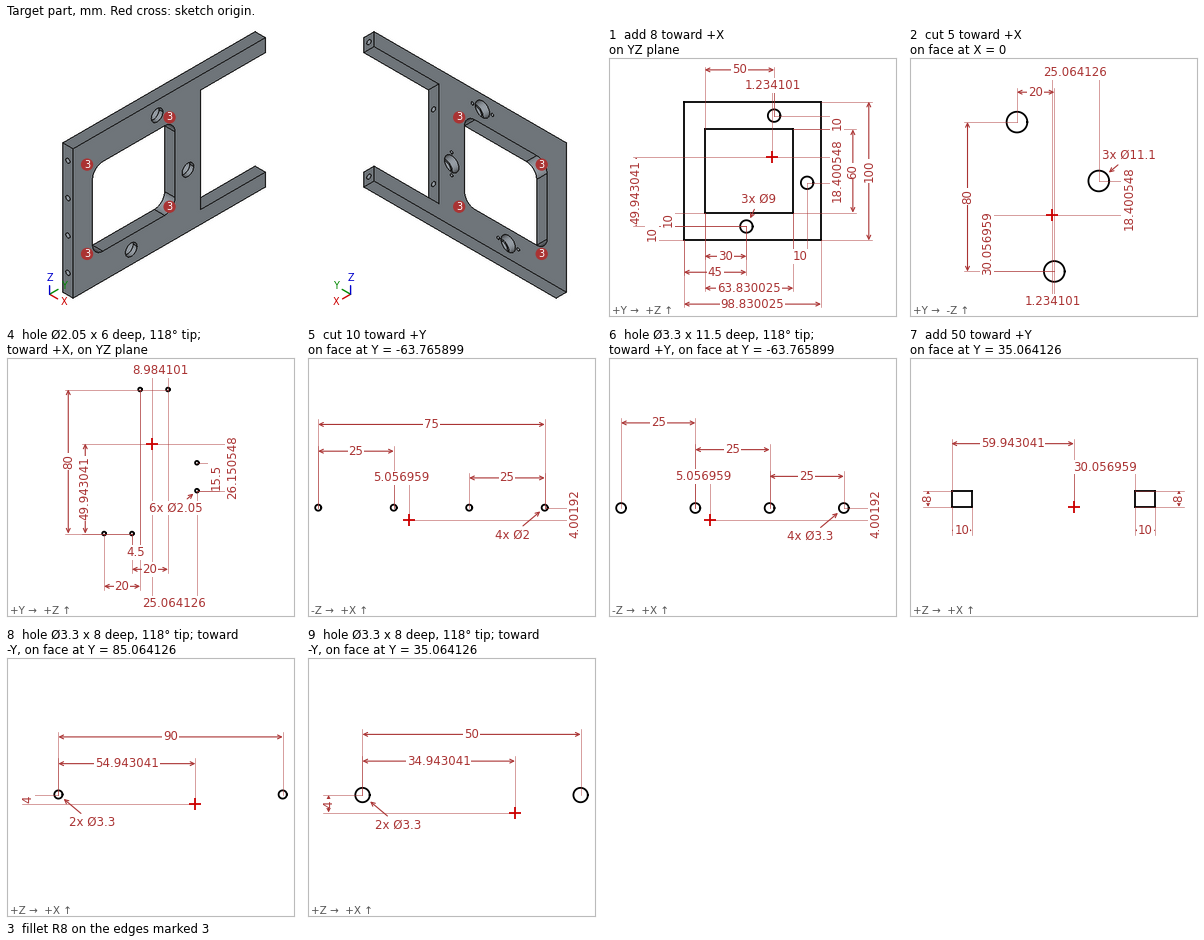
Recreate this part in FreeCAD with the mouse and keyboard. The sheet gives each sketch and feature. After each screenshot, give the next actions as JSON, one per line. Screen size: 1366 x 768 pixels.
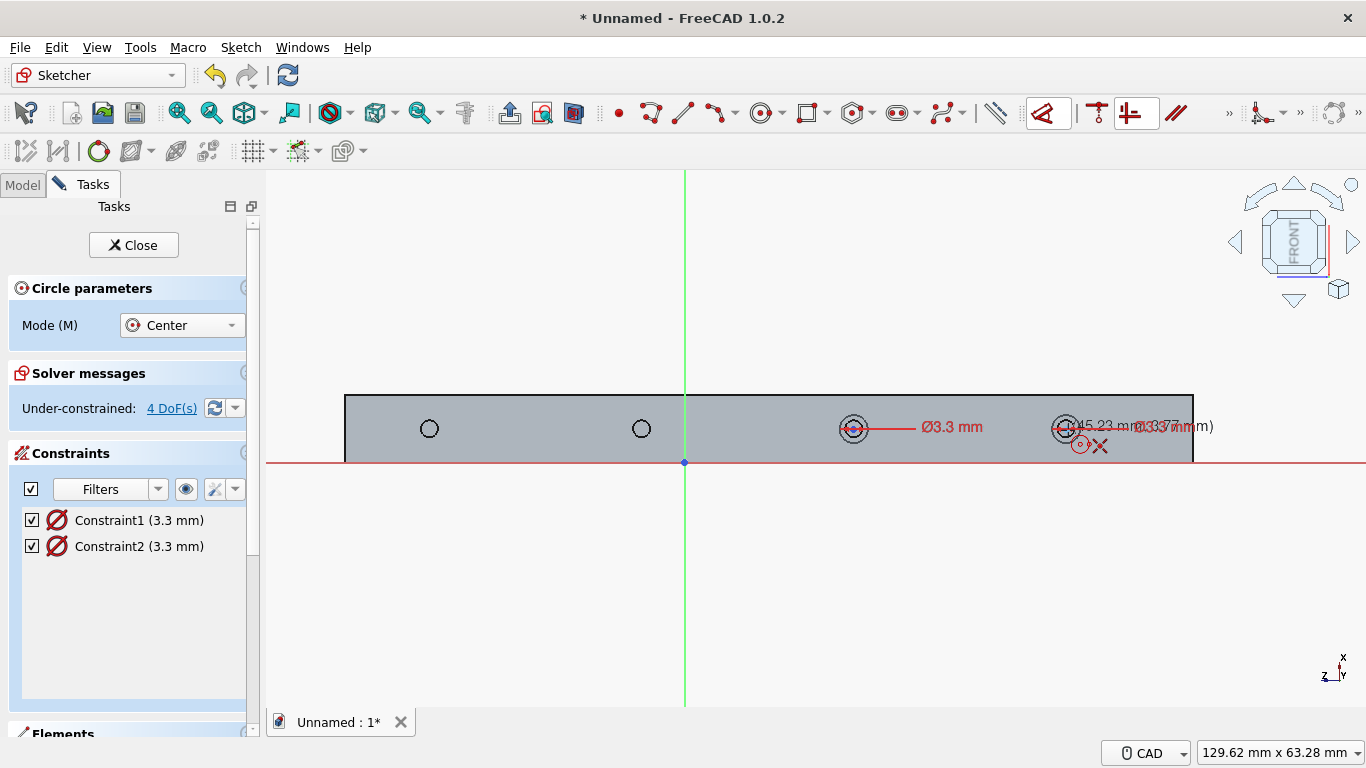
{"action": "scroll", "coordinate": [642, 429], "scroll_direction": "up", "scroll_amount": 3}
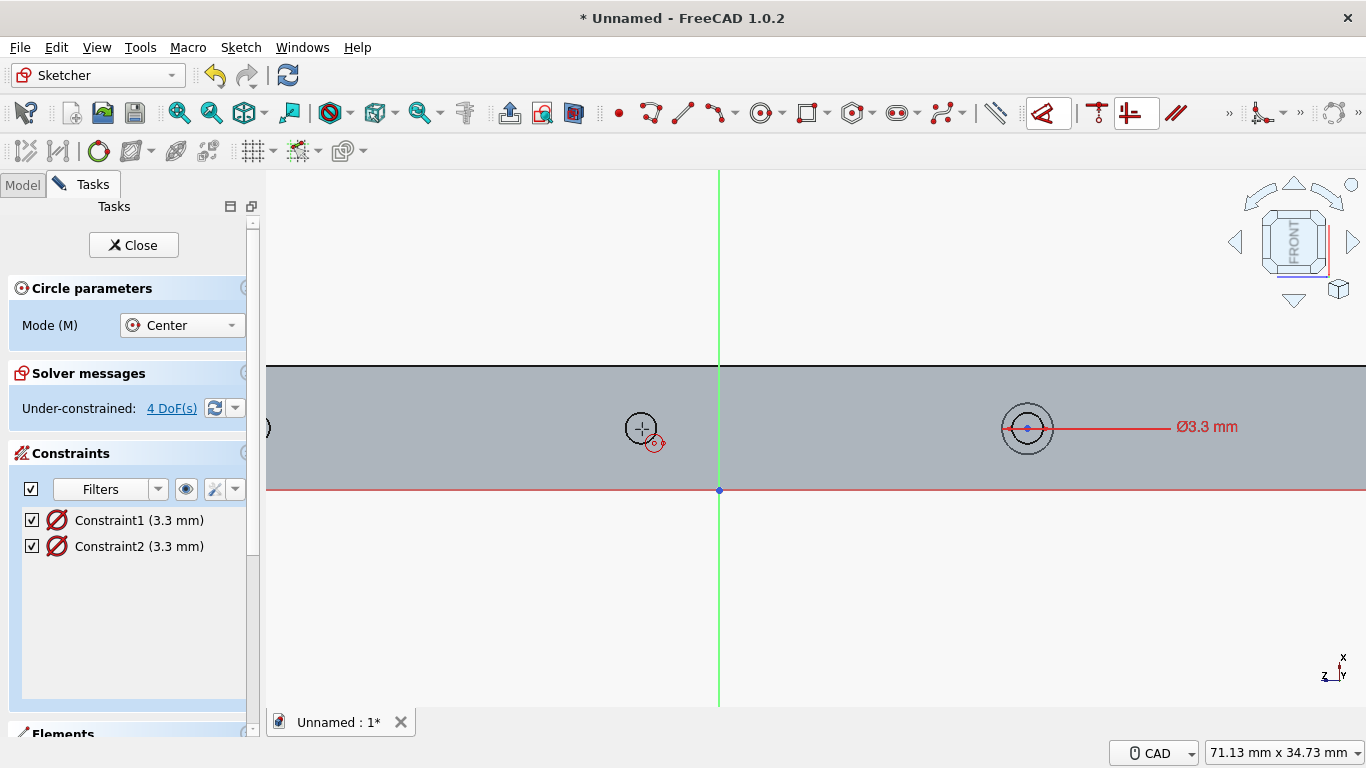
{"action": "left_click", "coordinate": [641, 428]}
{"action": "mouse_move", "coordinate": [659, 410]}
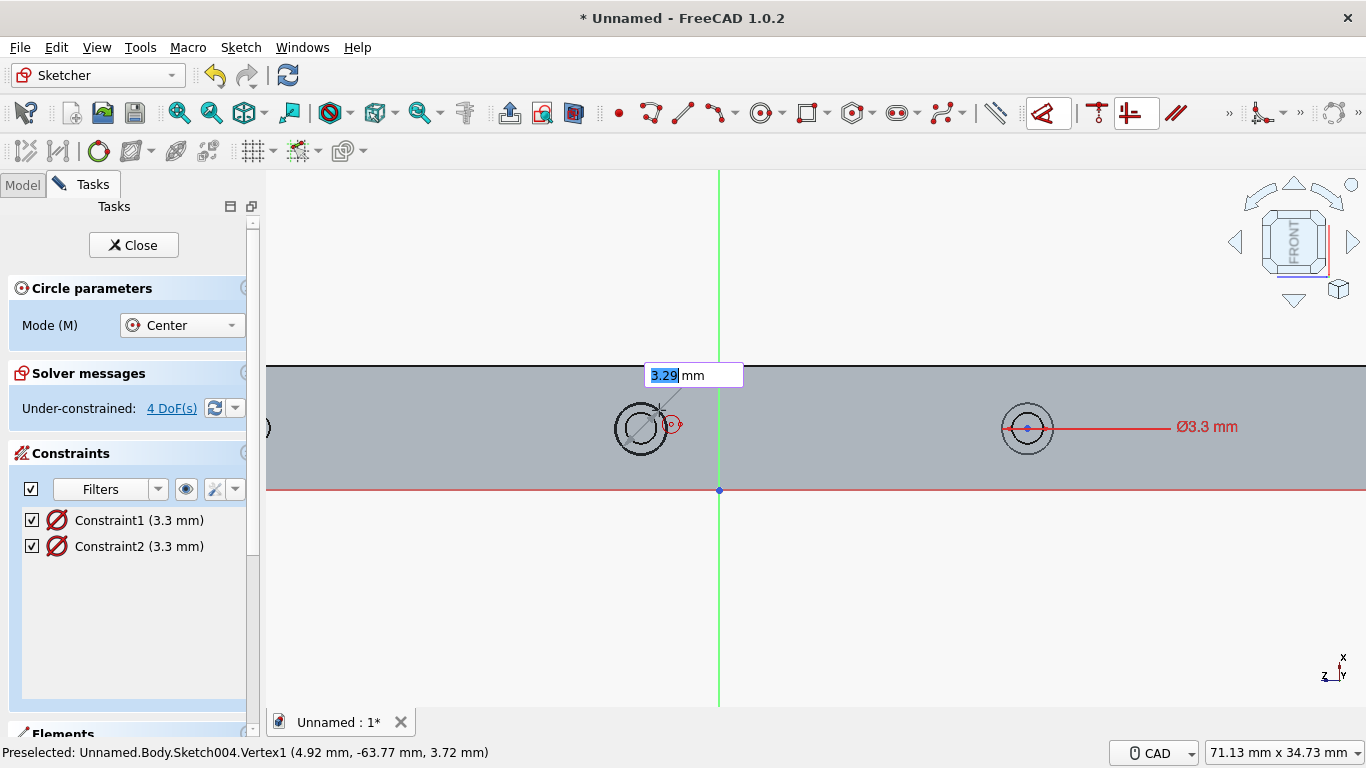
{"action": "type", "text": "3.3"}
{"action": "key", "text": "Return"}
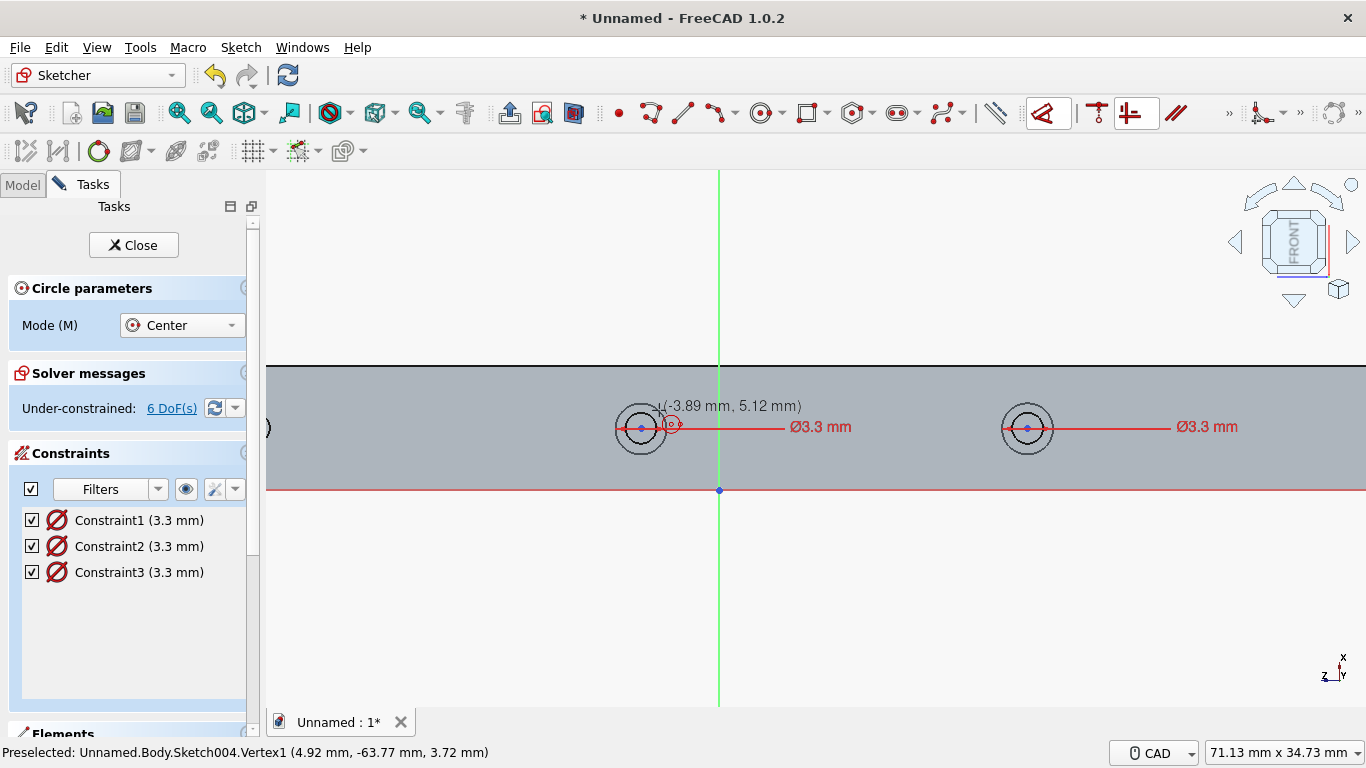
{"action": "scroll", "coordinate": [642, 429], "scroll_direction": "down", "scroll_amount": 3}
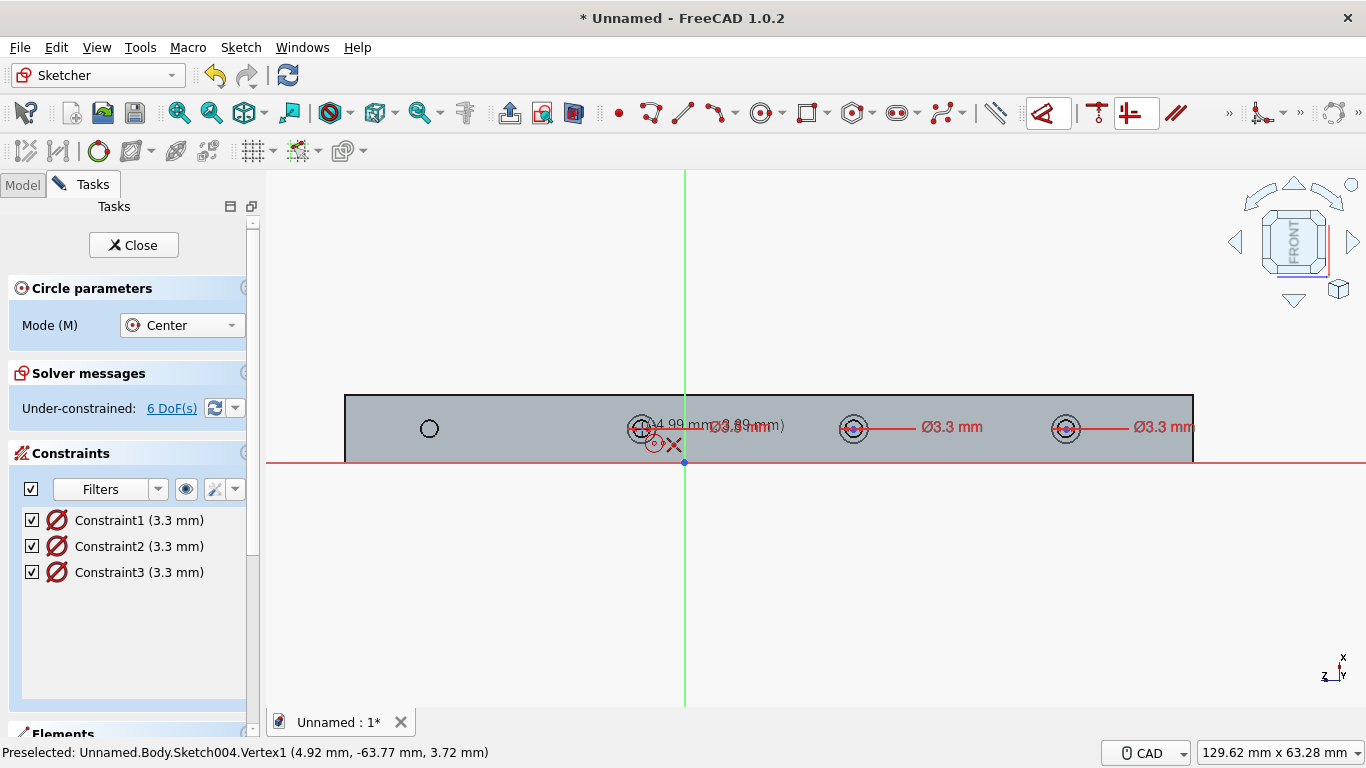
{"action": "scroll", "coordinate": [429, 429], "scroll_direction": "up", "scroll_amount": 3}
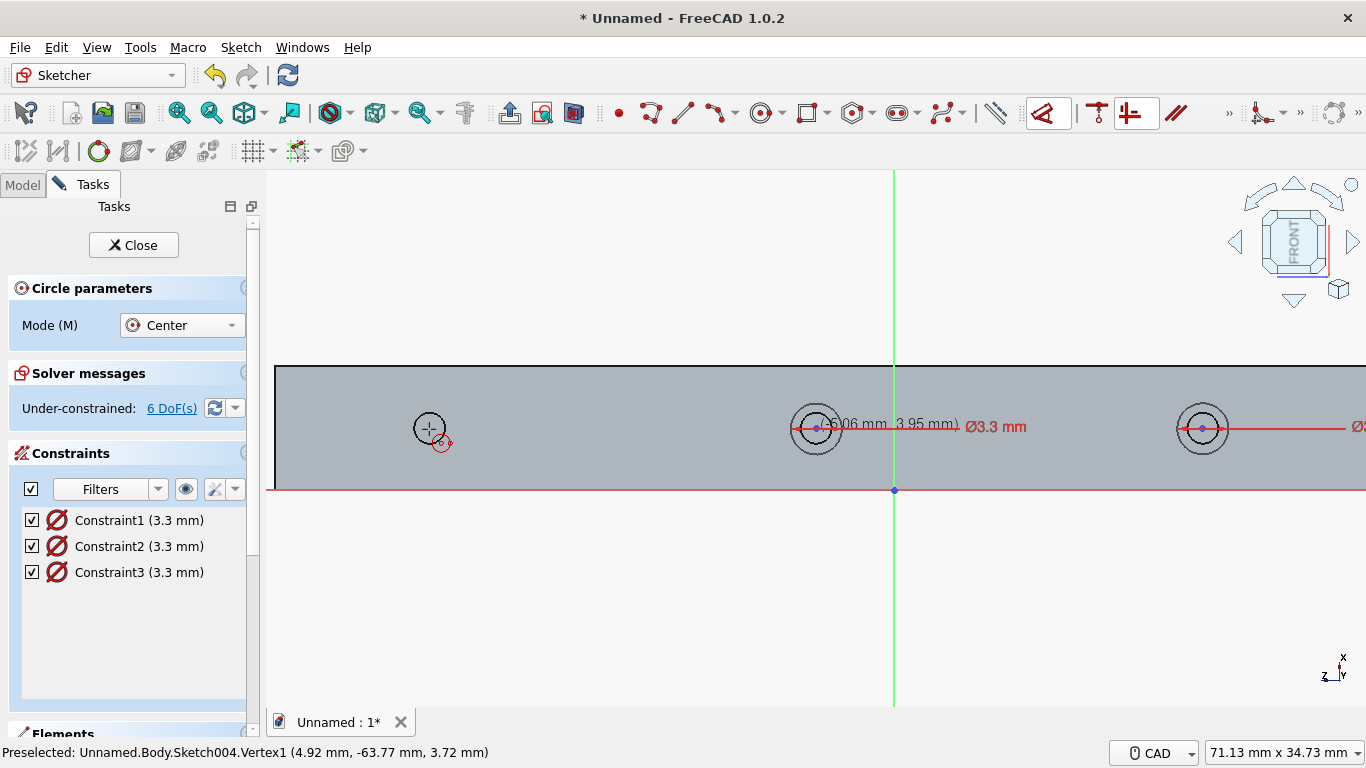
{"action": "left_click", "coordinate": [430, 428]}
{"action": "mouse_move", "coordinate": [448, 410]}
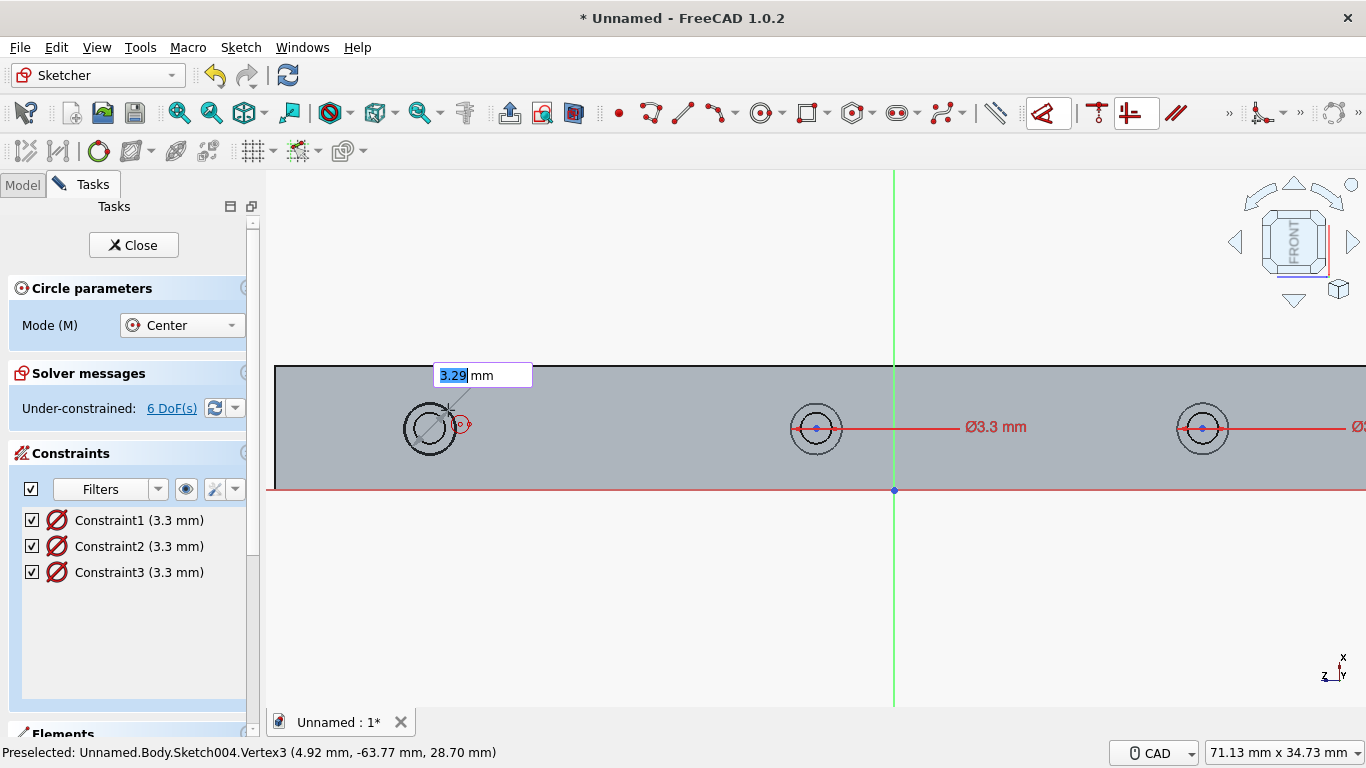
{"action": "type", "text": "3.3"}
{"action": "key", "text": "Return"}
{"action": "key", "text": "Escape"}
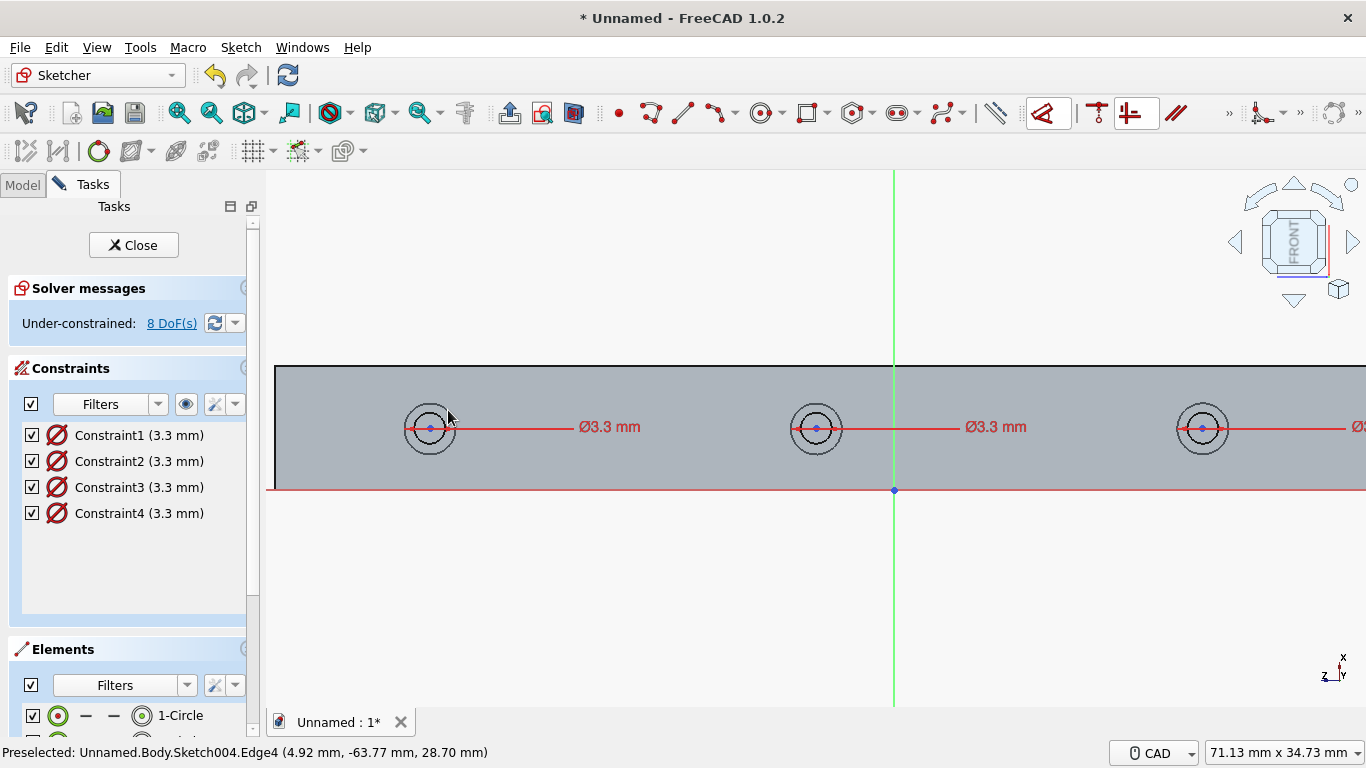
{"action": "scroll", "coordinate": [429, 429], "scroll_direction": "down", "scroll_amount": 3}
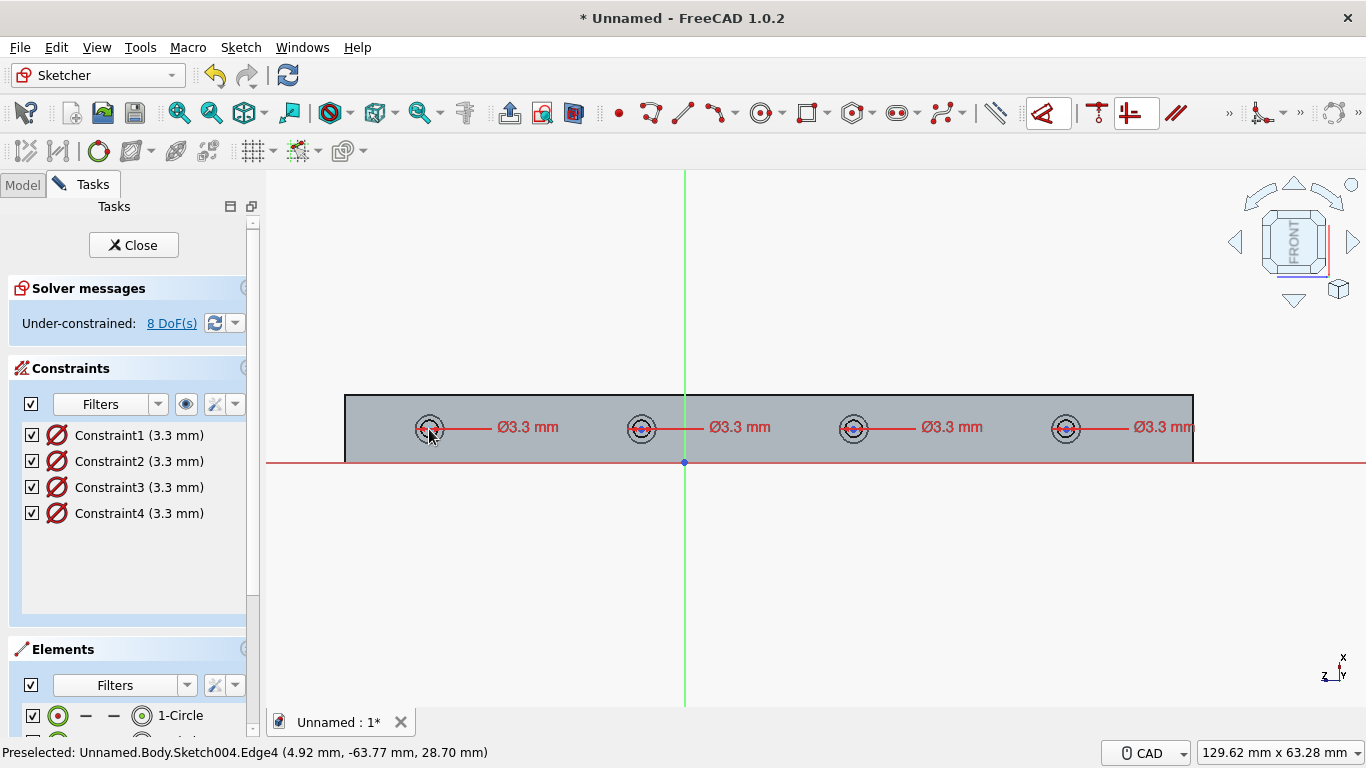
{"action": "left_click", "coordinate": [1066, 429]}